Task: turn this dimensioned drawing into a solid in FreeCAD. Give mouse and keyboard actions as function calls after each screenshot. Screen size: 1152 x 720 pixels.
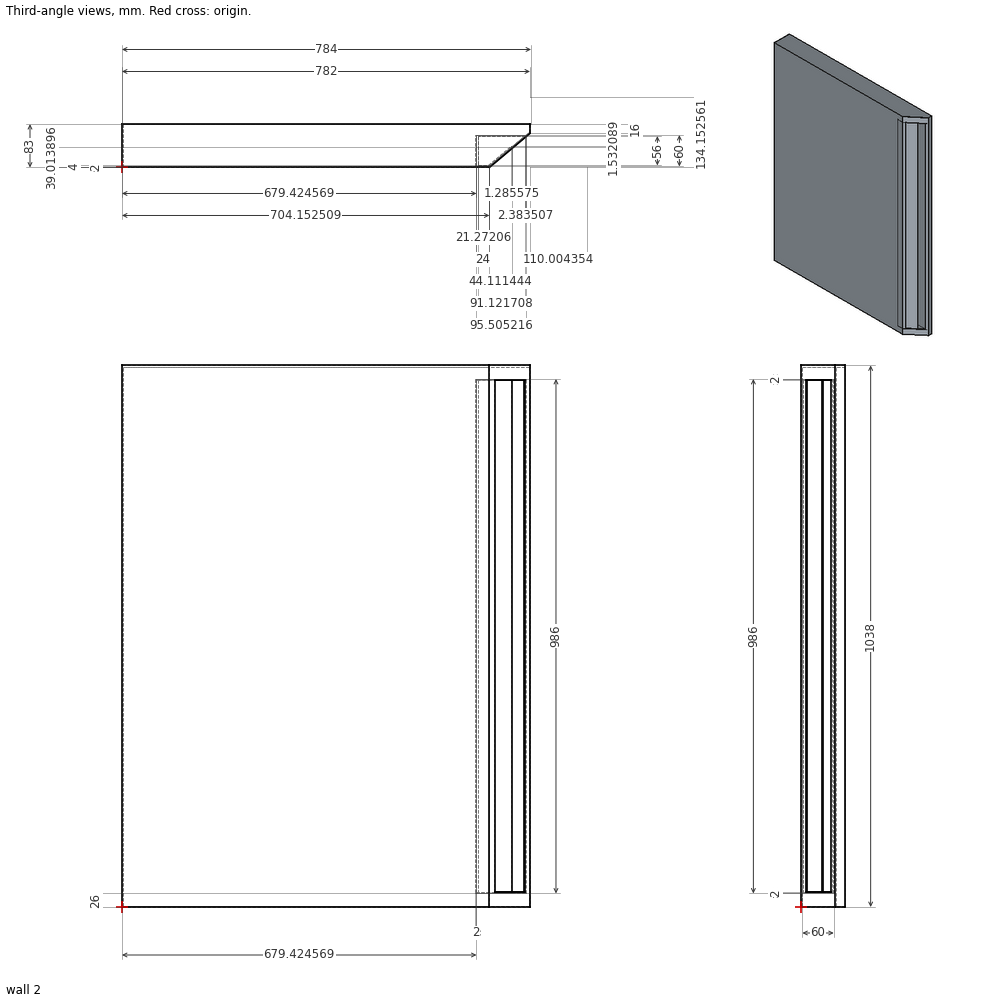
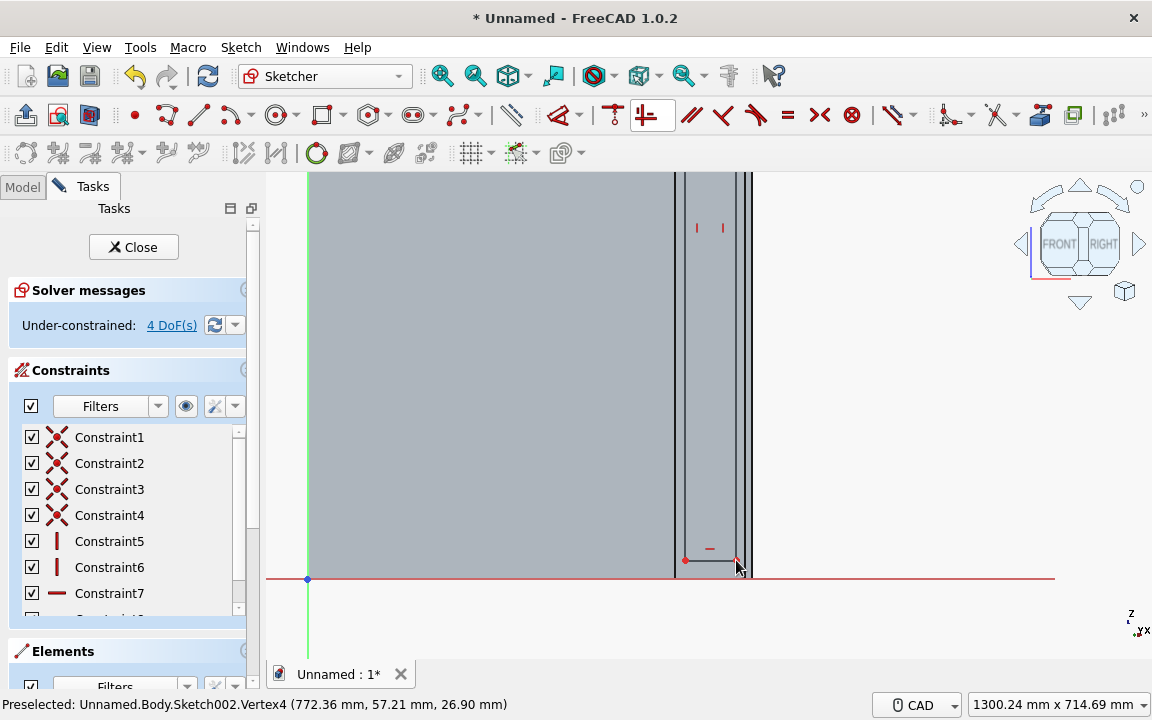
key(d)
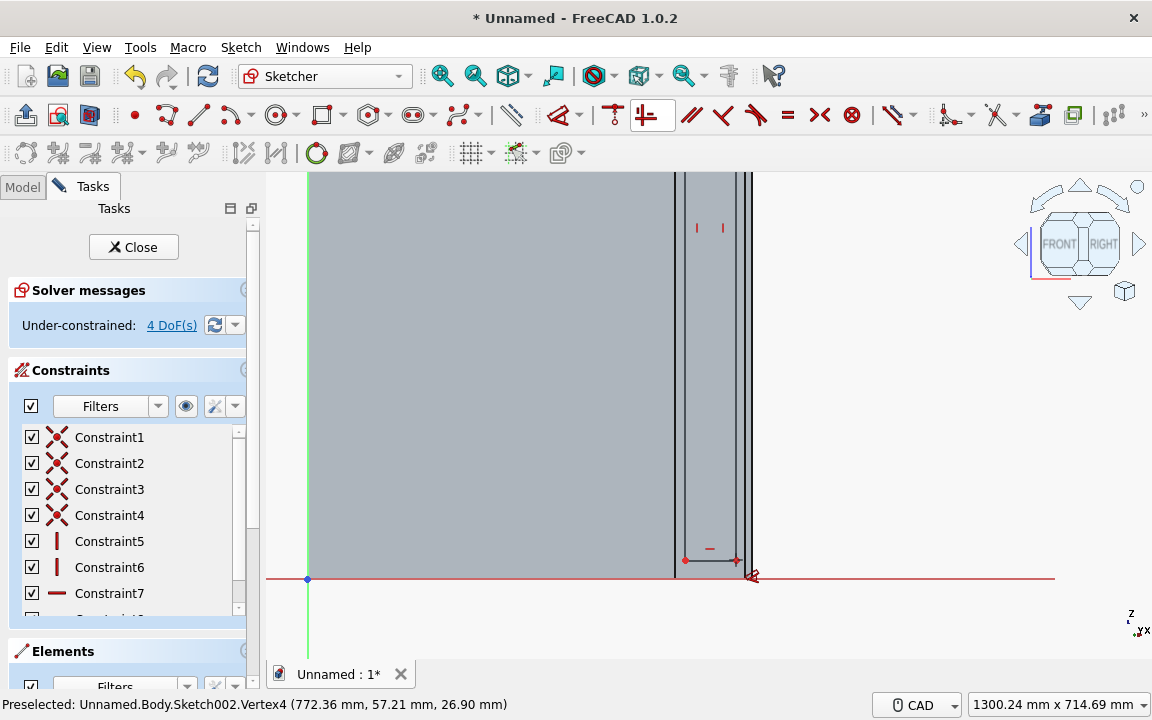
click(700, 561)
click(711, 595)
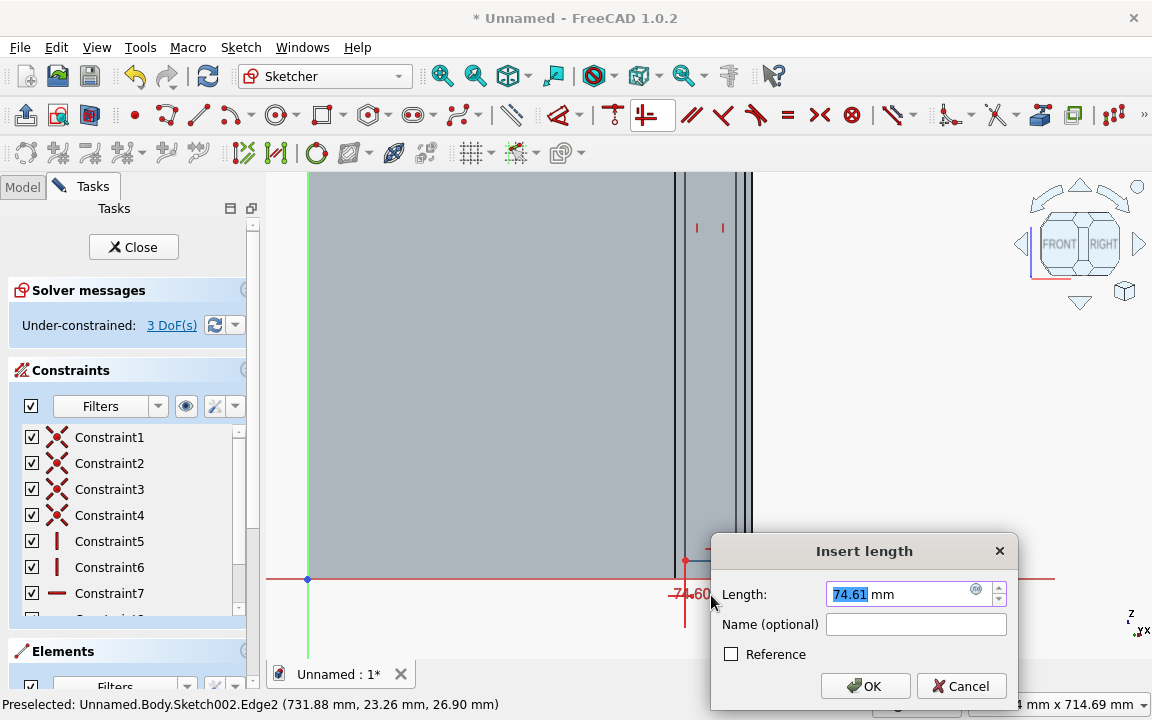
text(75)
key(Return)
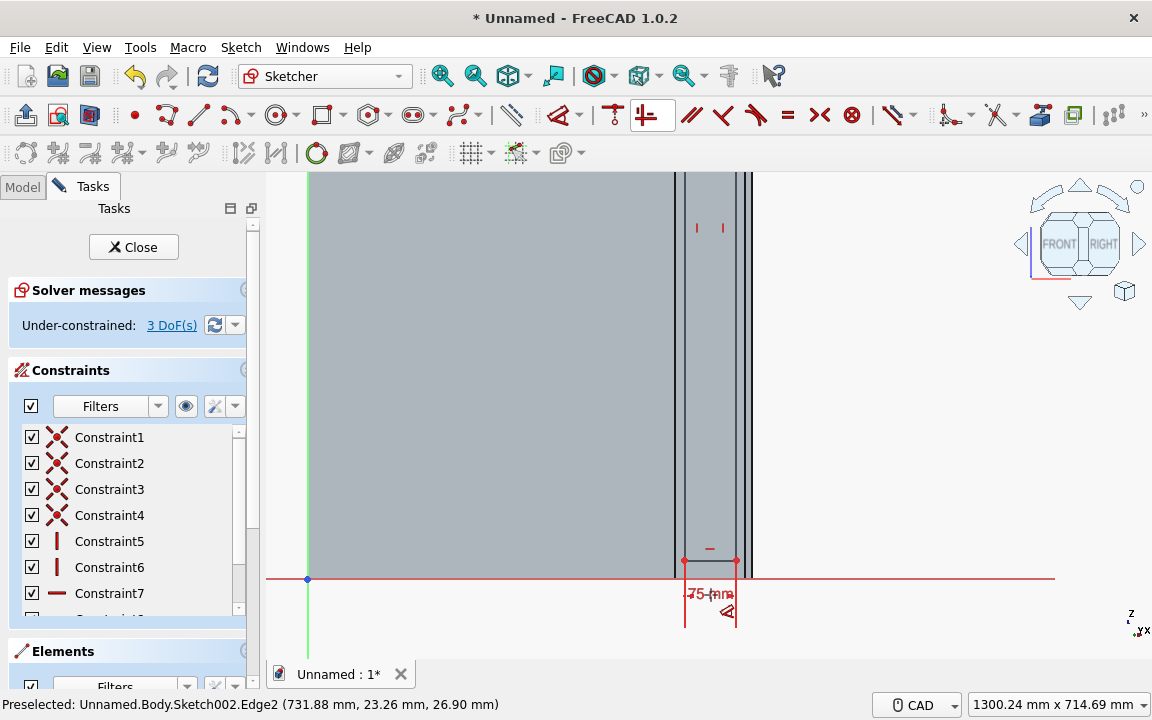
click(685, 361)
click(719, 381)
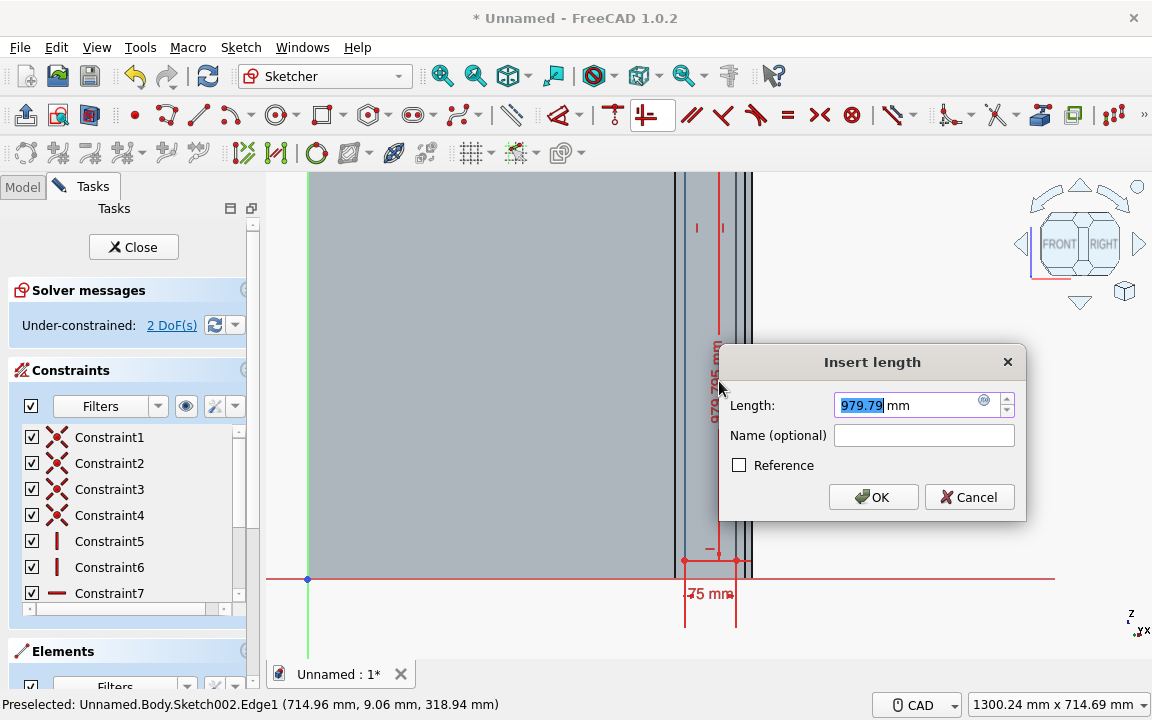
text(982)
key(Return)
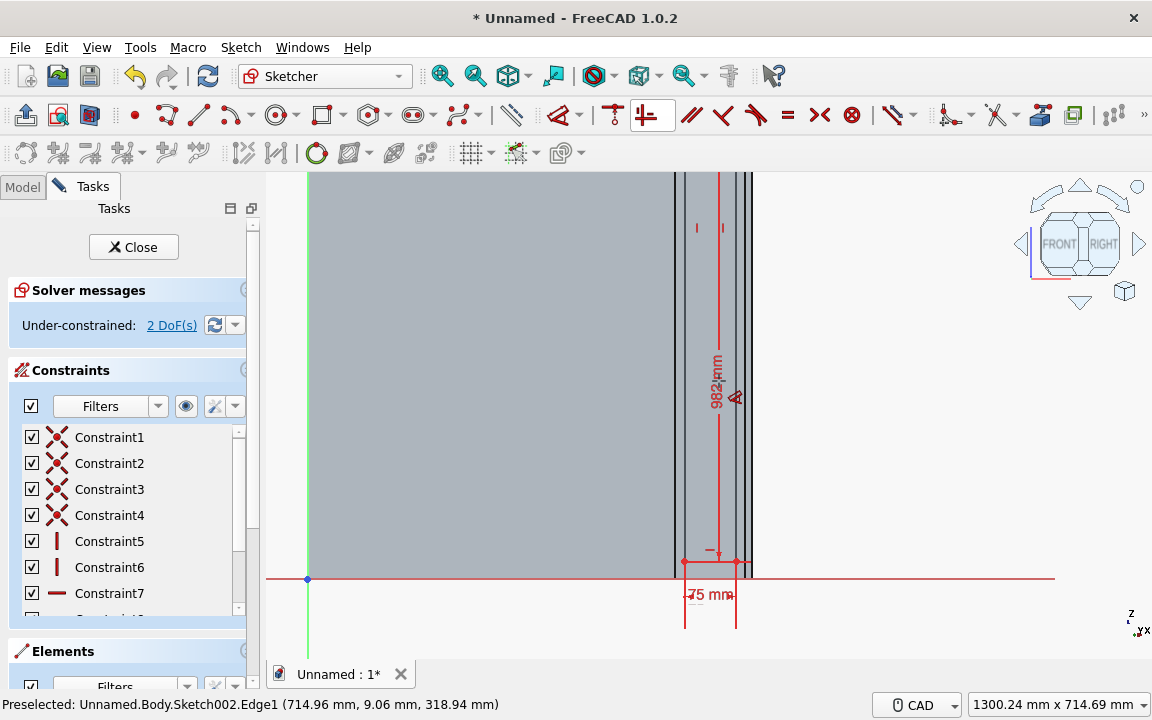
scroll(685, 562, up, 4)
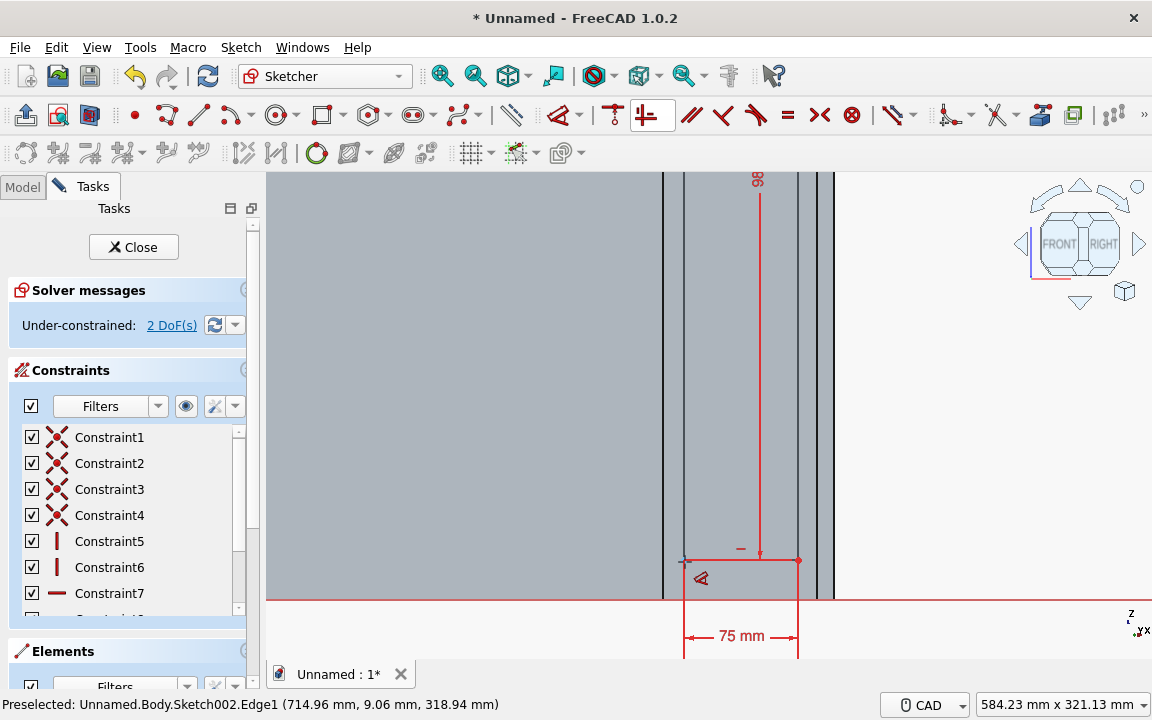
click(684, 560)
click(718, 580)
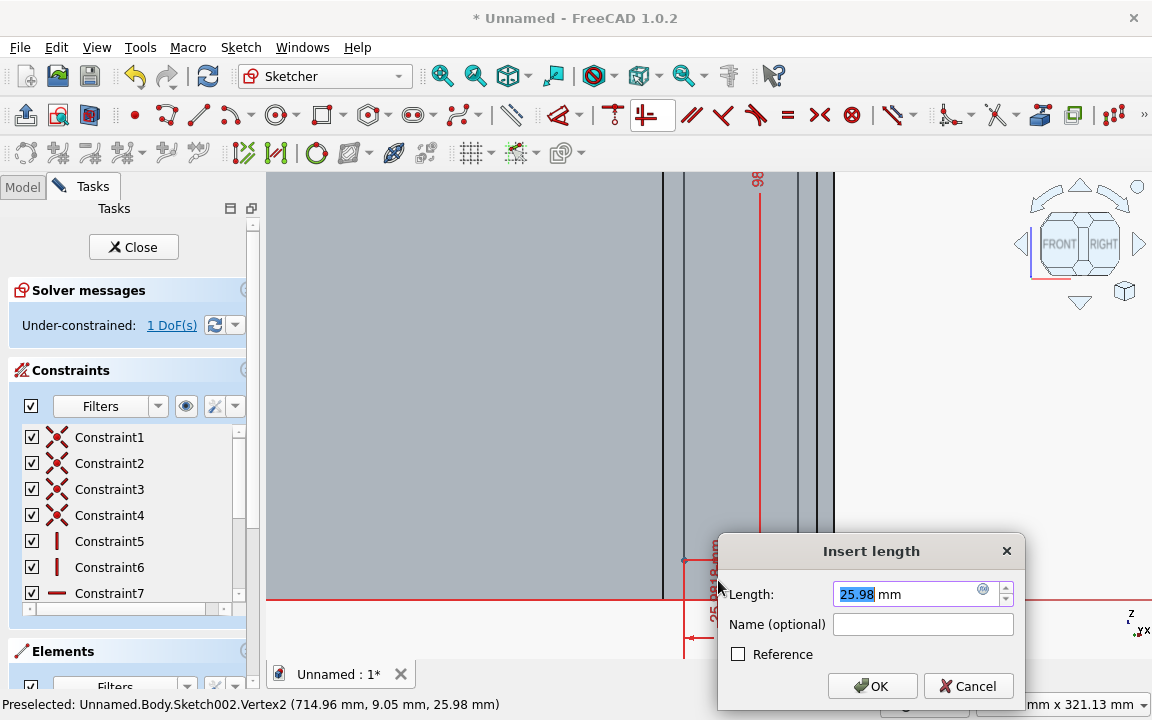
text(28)
key(Return)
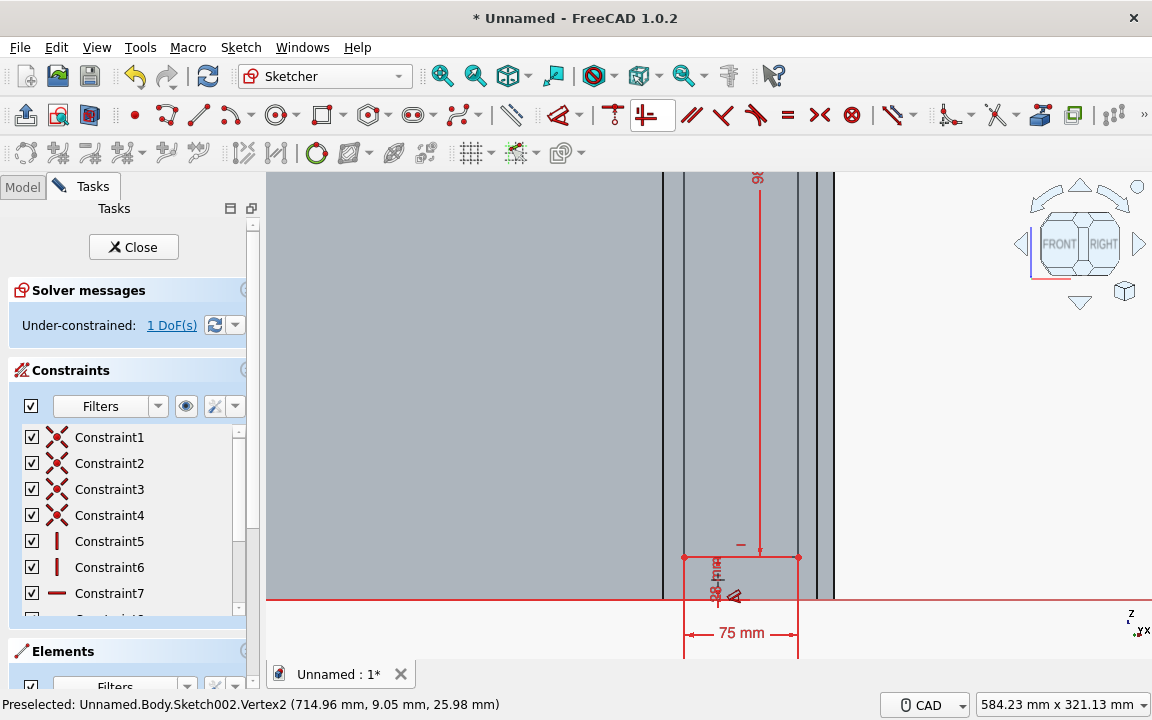
scroll(721, 563, down, 8)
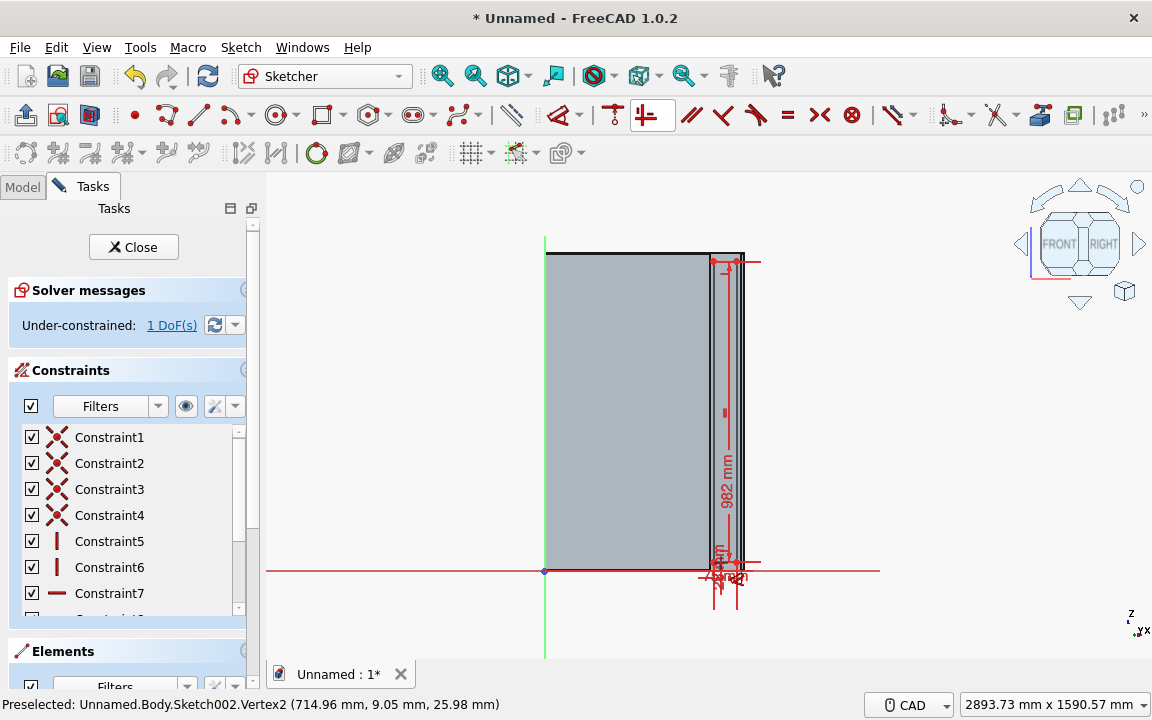
click(714, 262)
click(629, 605)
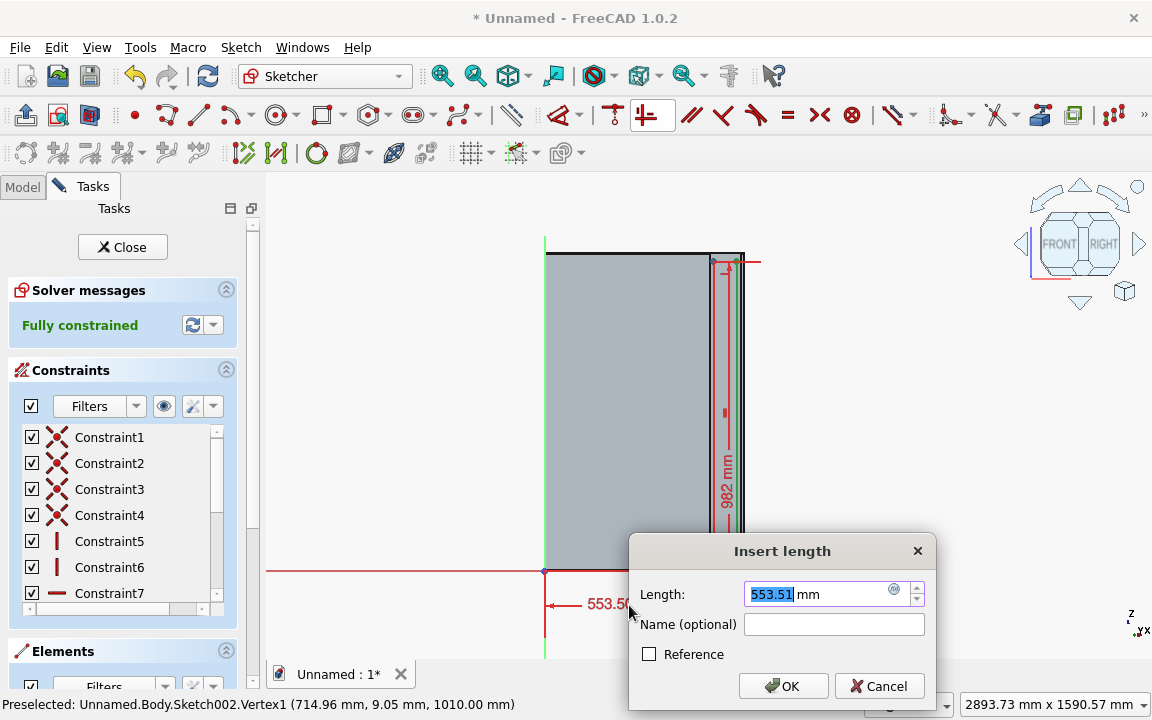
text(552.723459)
key(Return)
key(Escape)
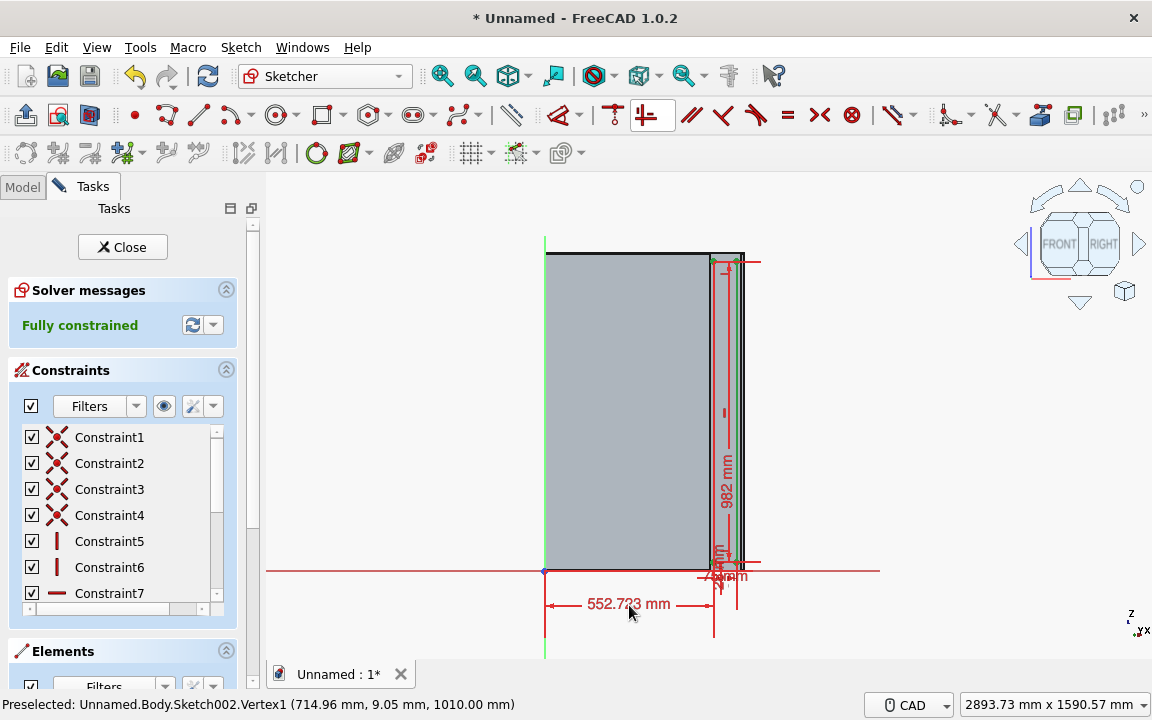
click(123, 247)